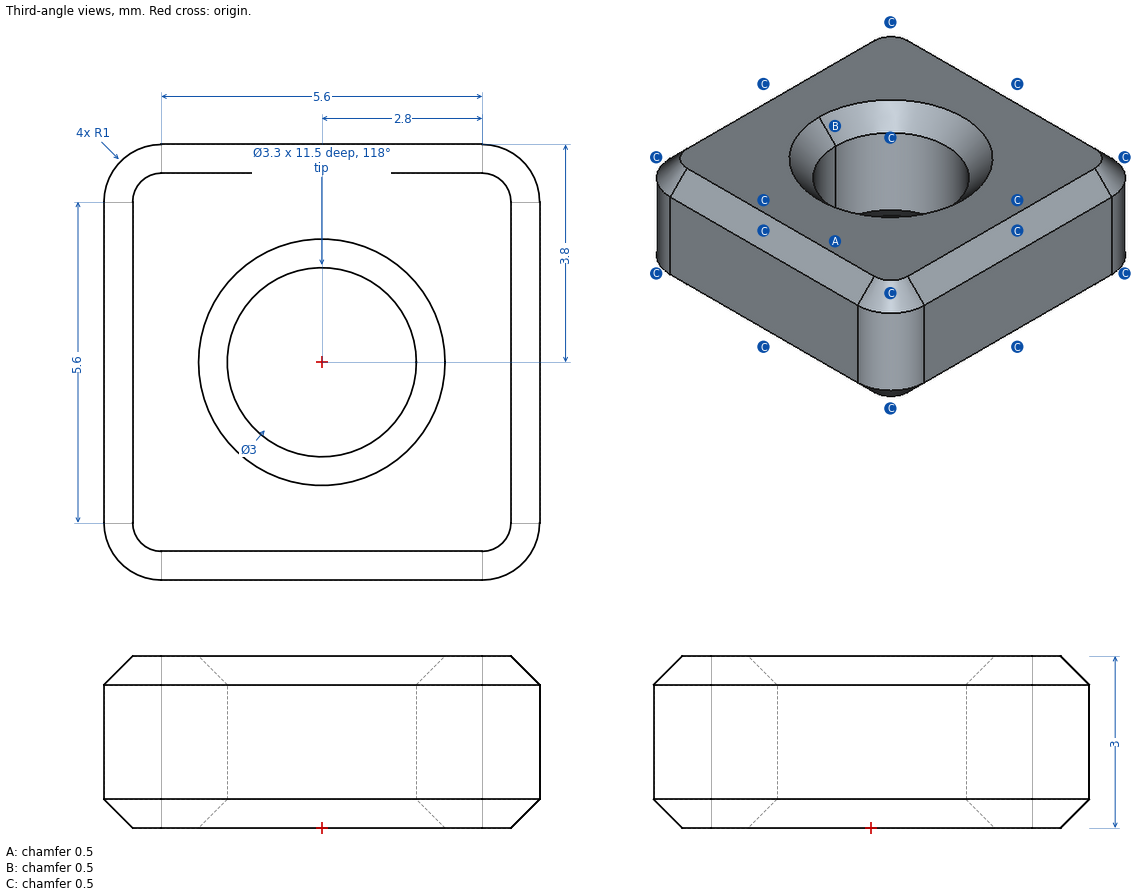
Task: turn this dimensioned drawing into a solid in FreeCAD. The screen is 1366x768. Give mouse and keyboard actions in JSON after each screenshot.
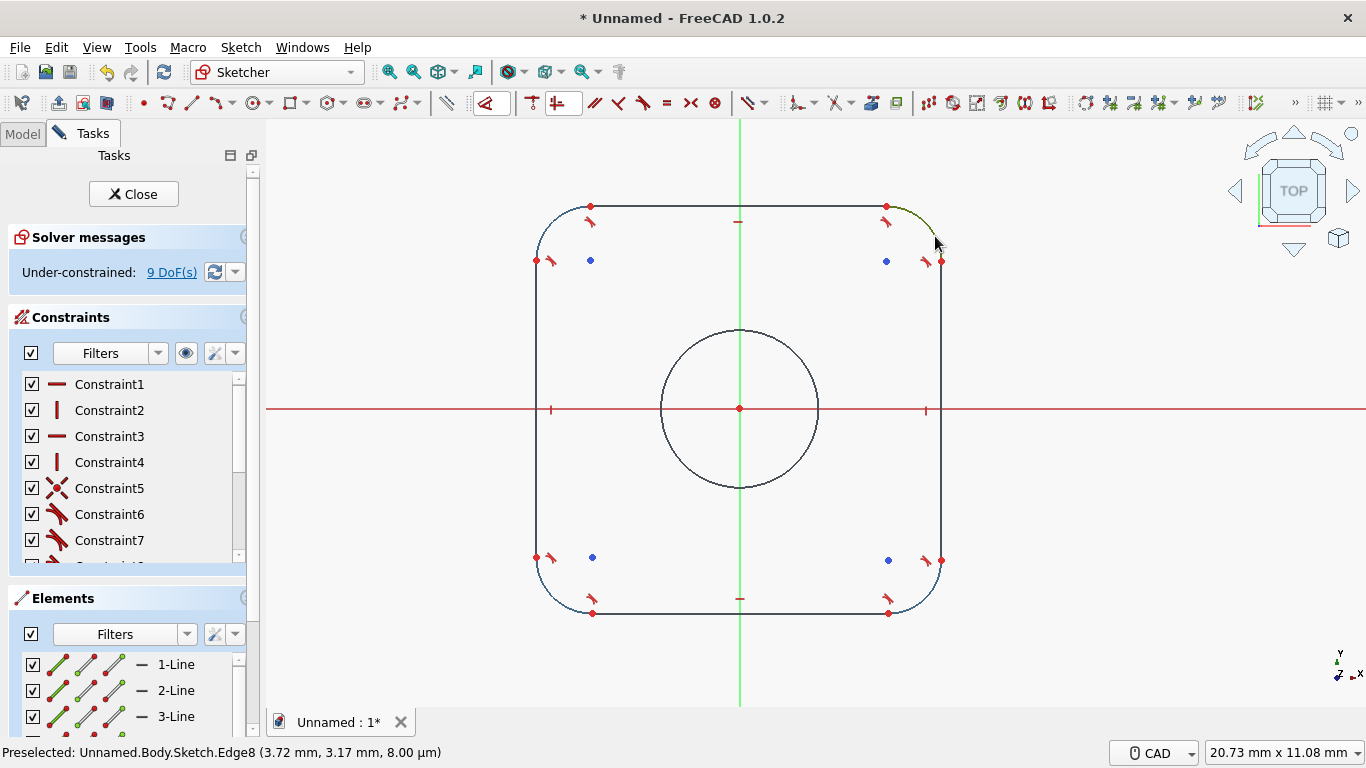
{"action": "key", "text": "e"}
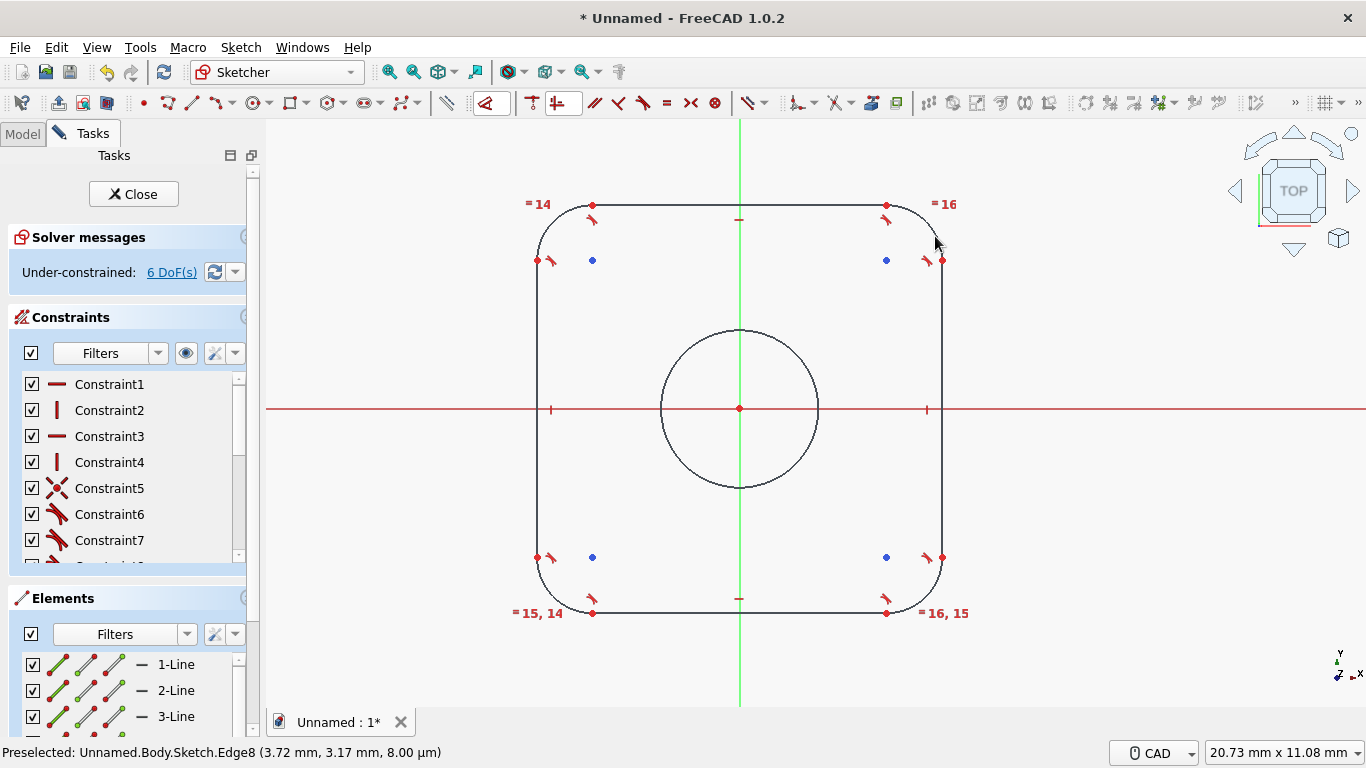
{"action": "key", "text": "d"}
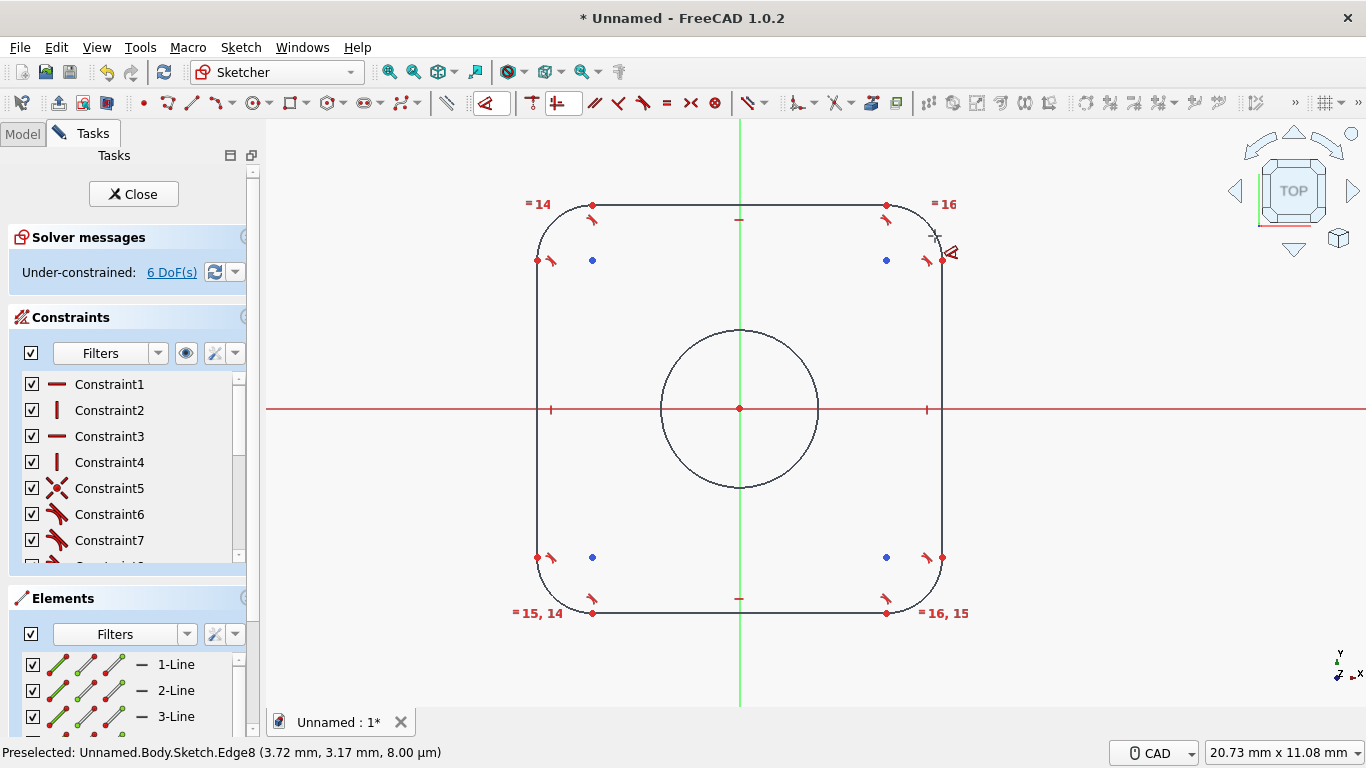
{"action": "left_click", "coordinate": [568, 211]}
{"action": "left_click", "coordinate": [554, 182]}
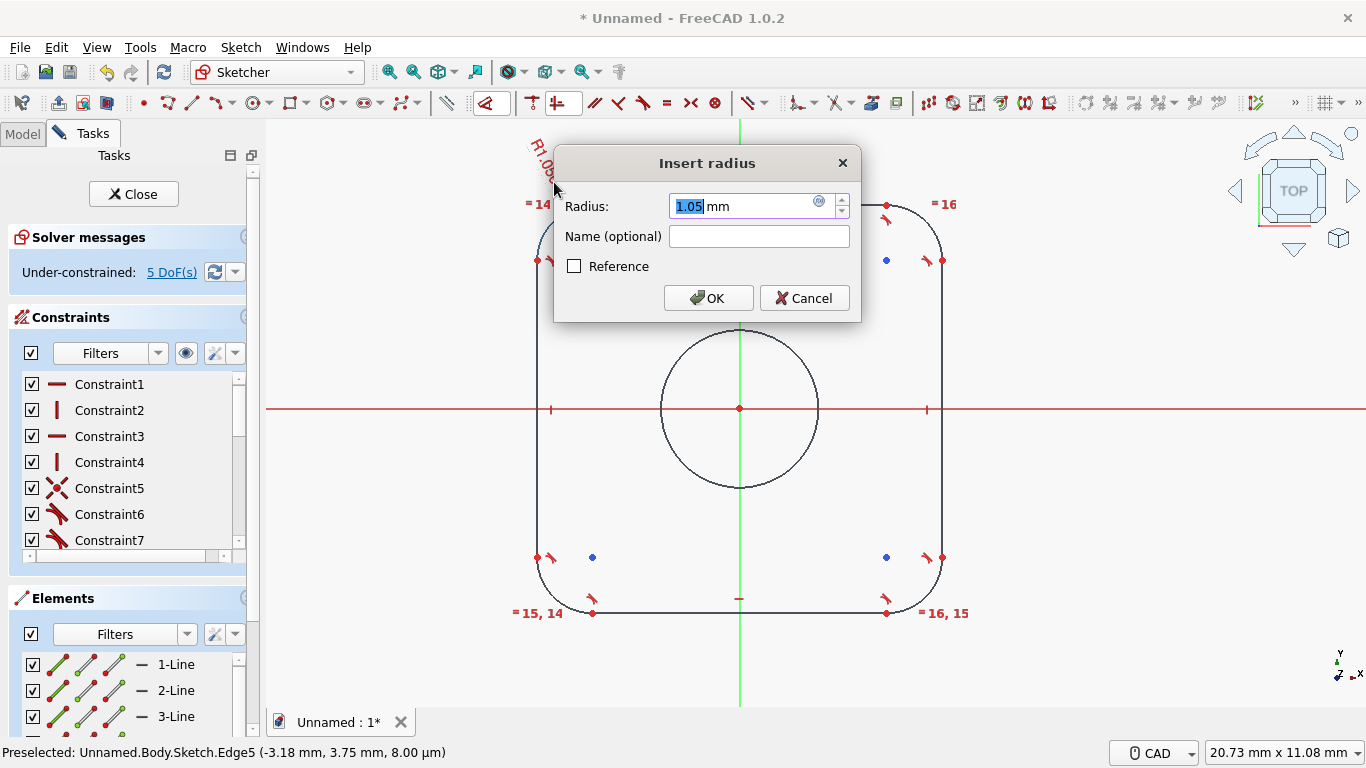
{"action": "type", "text": "1"}
{"action": "key", "text": "Return"}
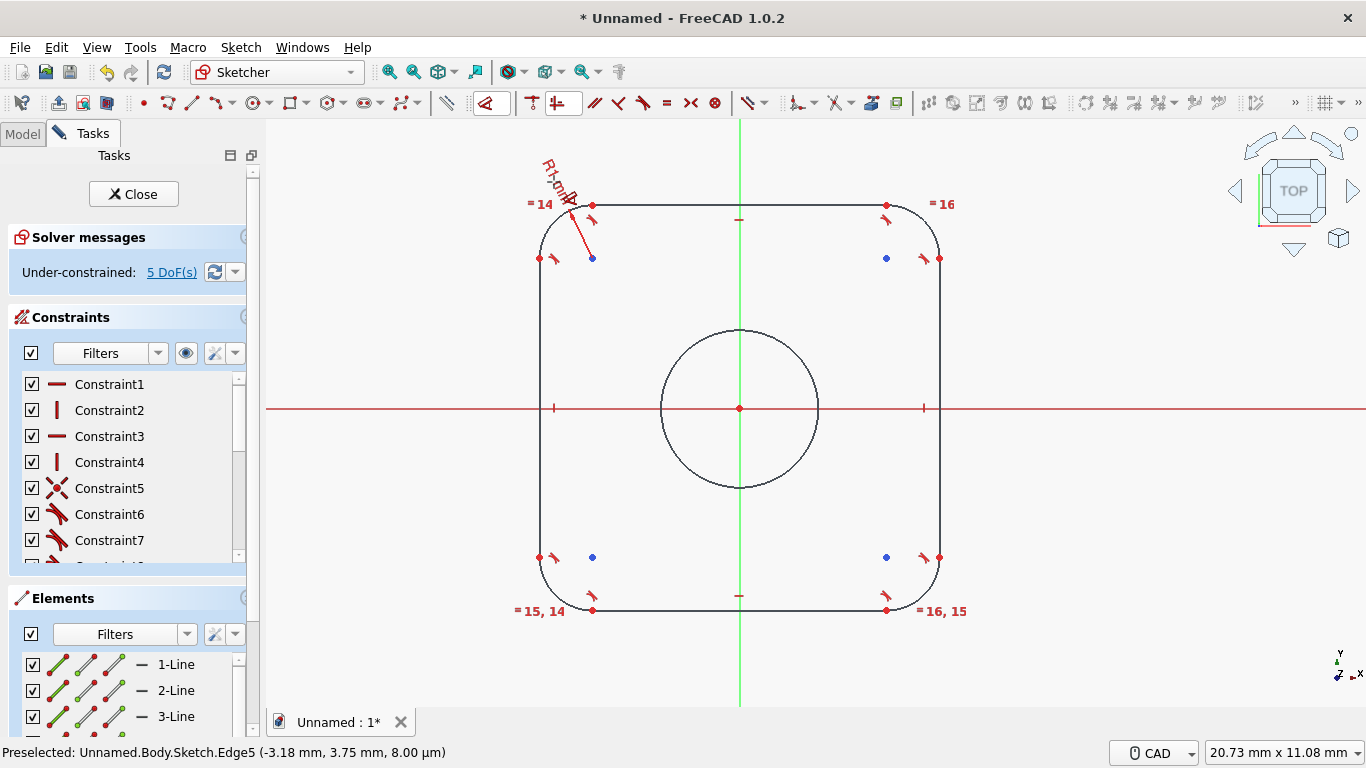
{"action": "left_click", "coordinate": [795, 353]}
{"action": "left_click", "coordinate": [817, 330]}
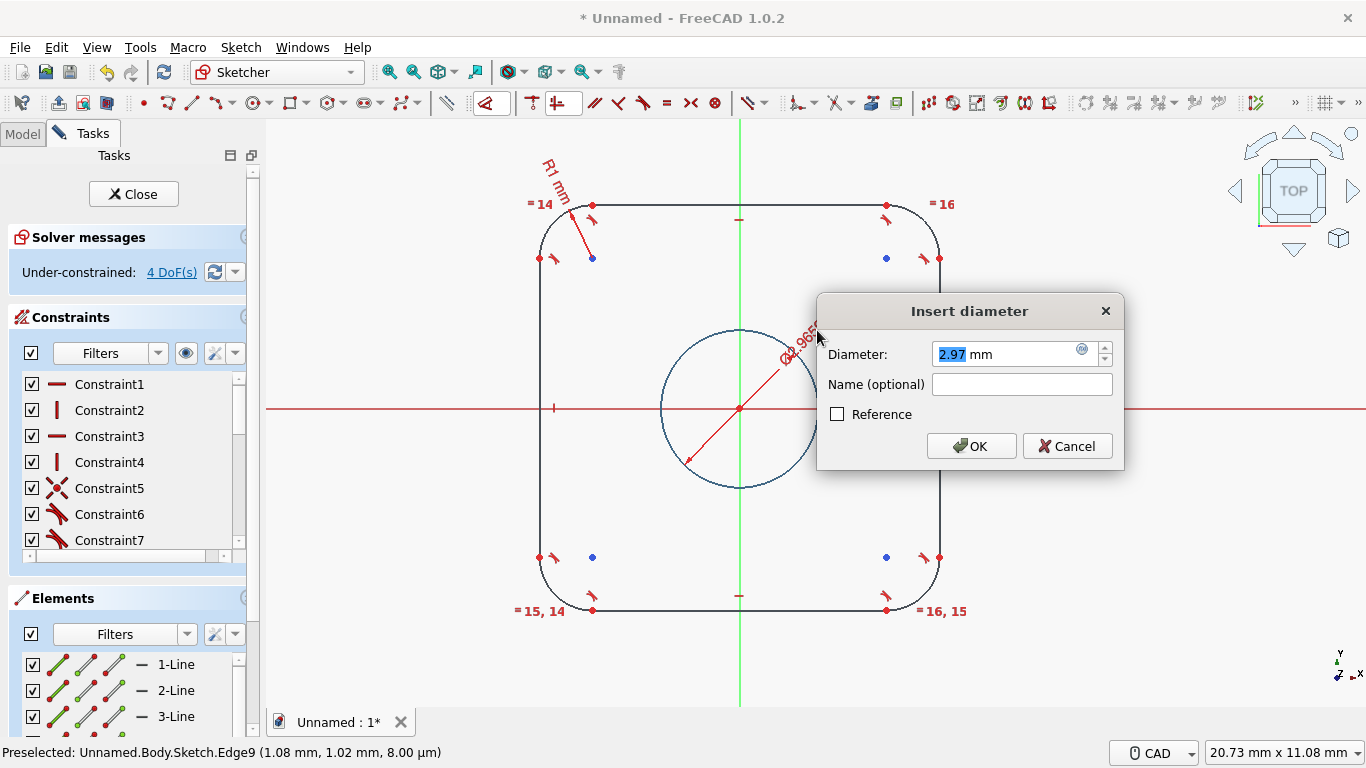
{"action": "type", "text": "3"}
{"action": "key", "text": "Return"}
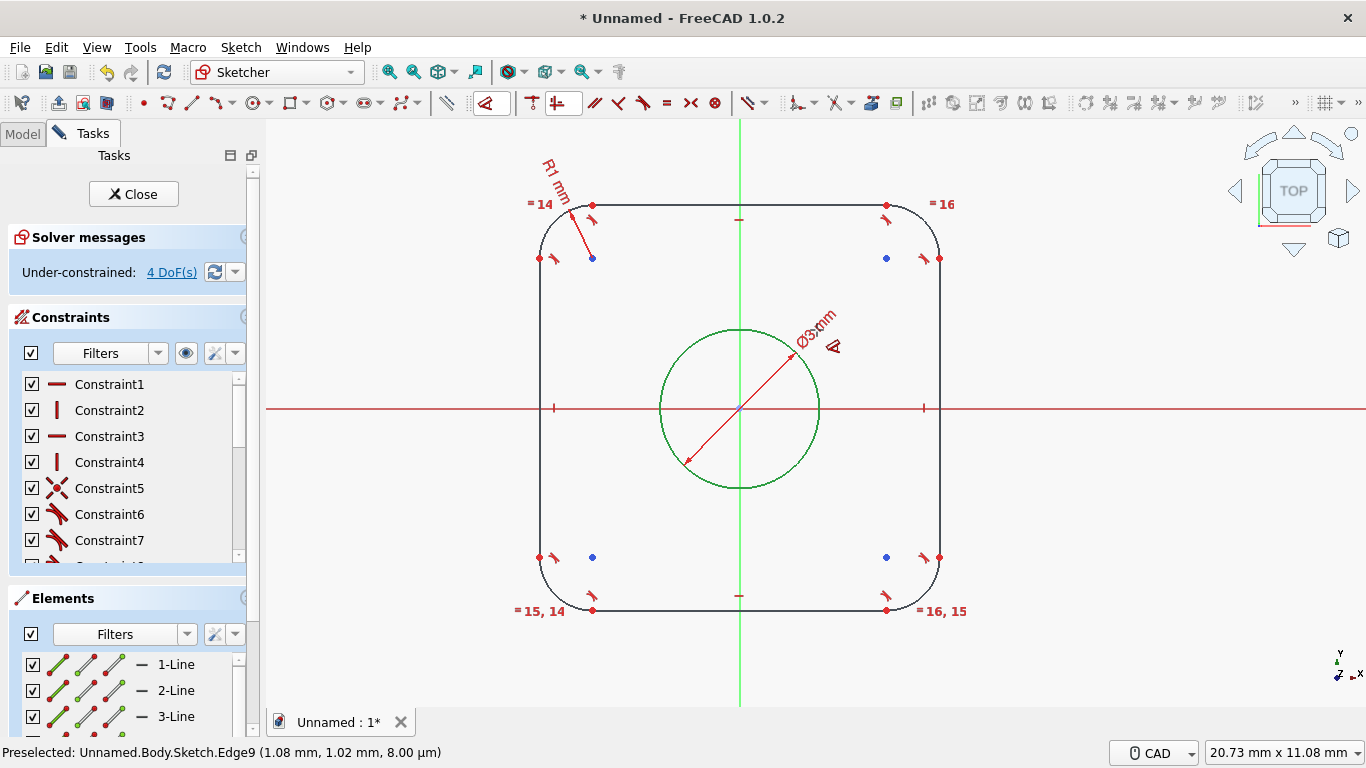
{"action": "left_click", "coordinate": [798, 205]}
{"action": "left_click", "coordinate": [672, 171]}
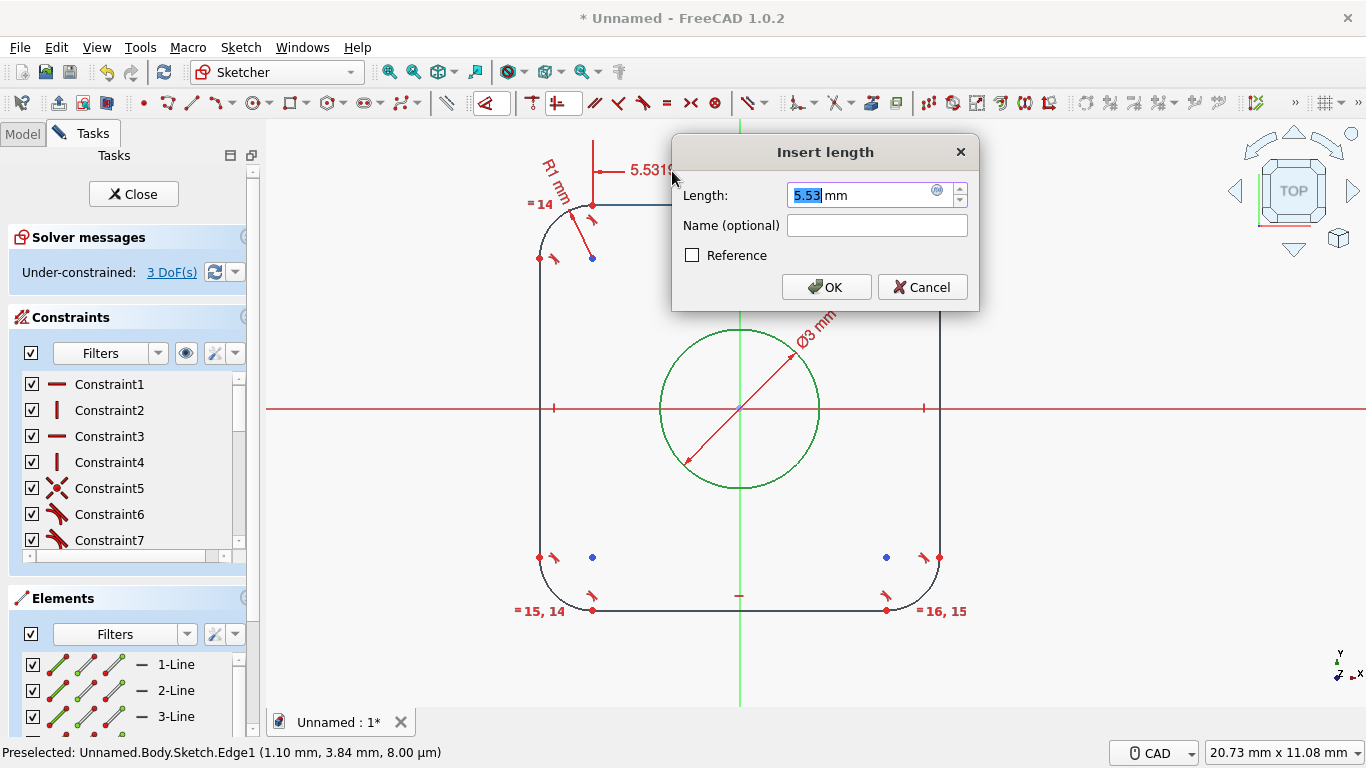
{"action": "type", "text": "5.6"}
{"action": "key", "text": "Return"}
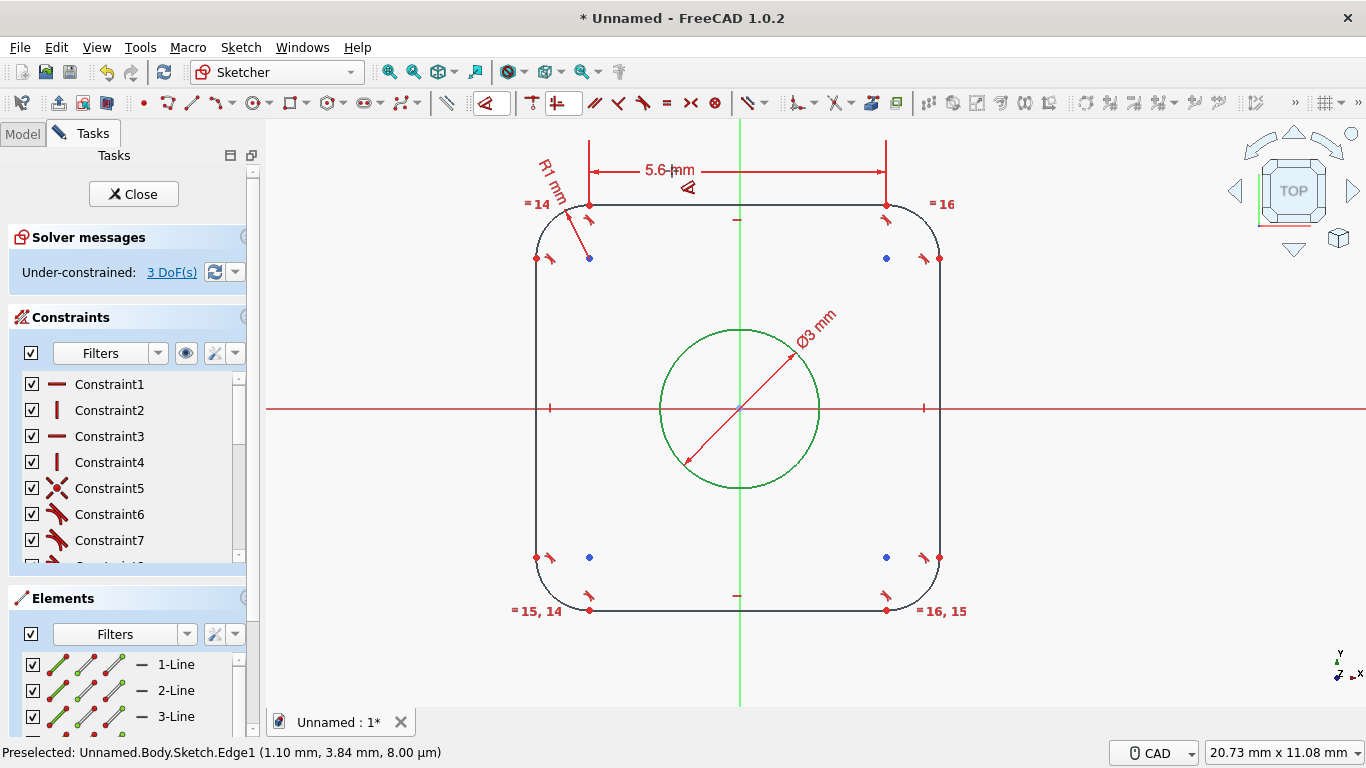
{"action": "left_click", "coordinate": [536, 348]}
{"action": "left_click", "coordinate": [502, 339]}